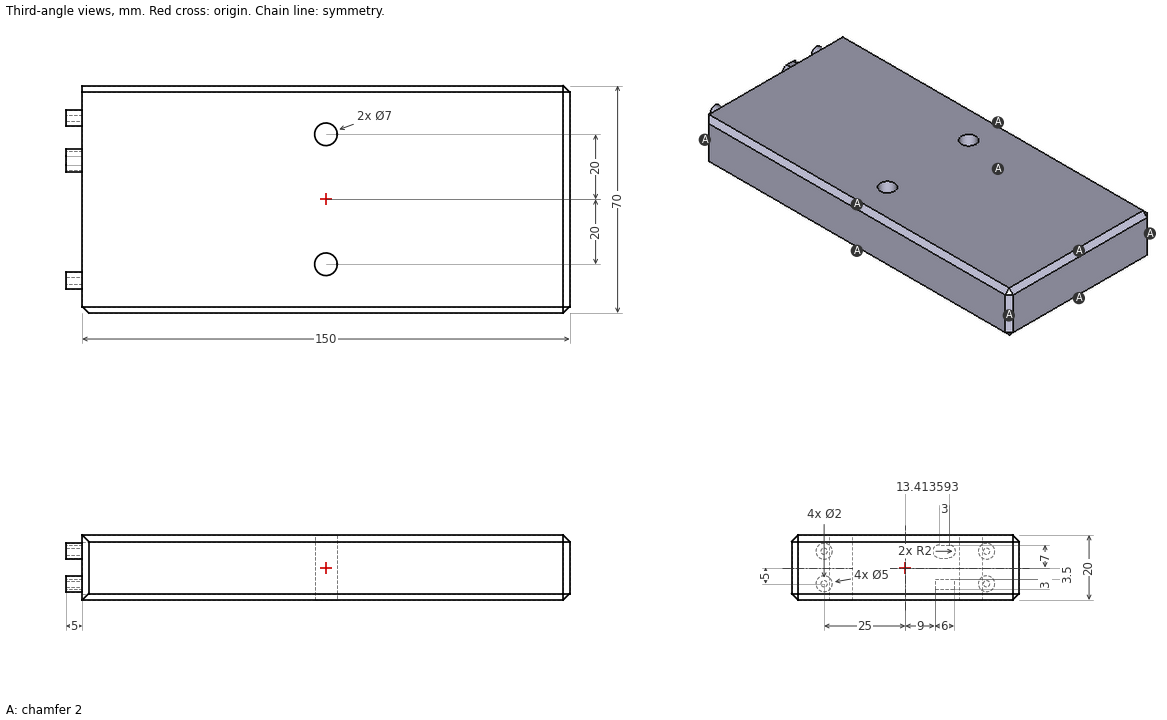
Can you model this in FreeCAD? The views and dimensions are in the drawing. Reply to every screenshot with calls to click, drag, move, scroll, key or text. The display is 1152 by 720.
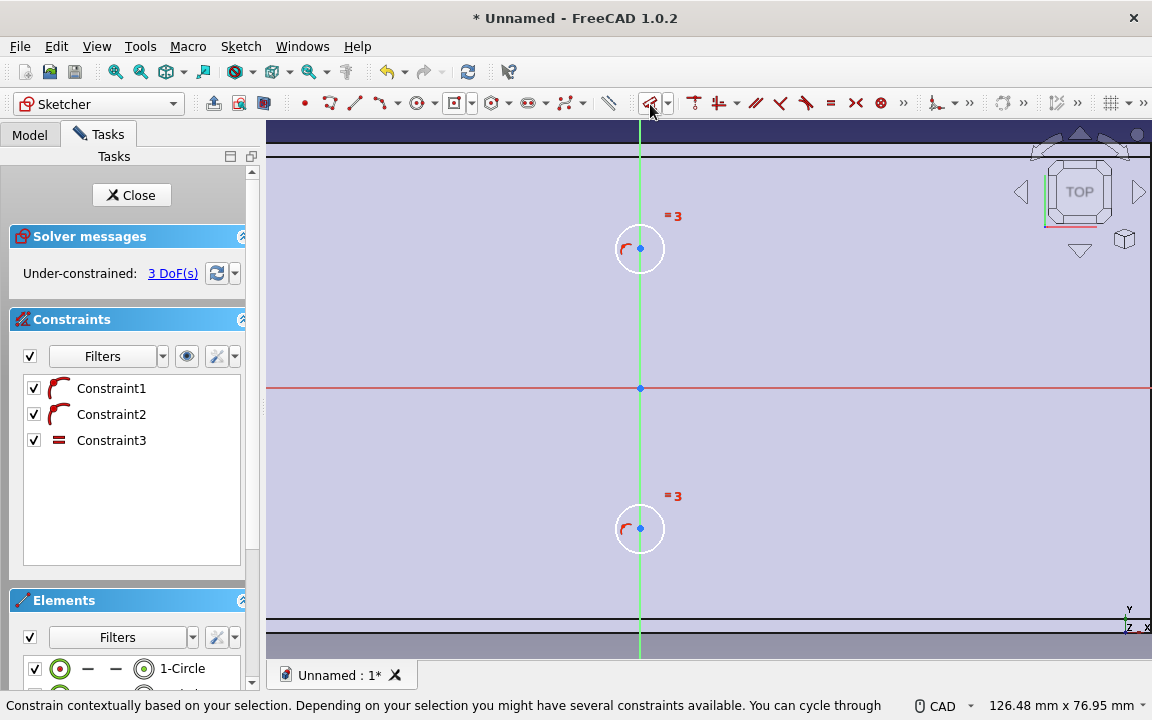
click(657, 232)
click(680, 209)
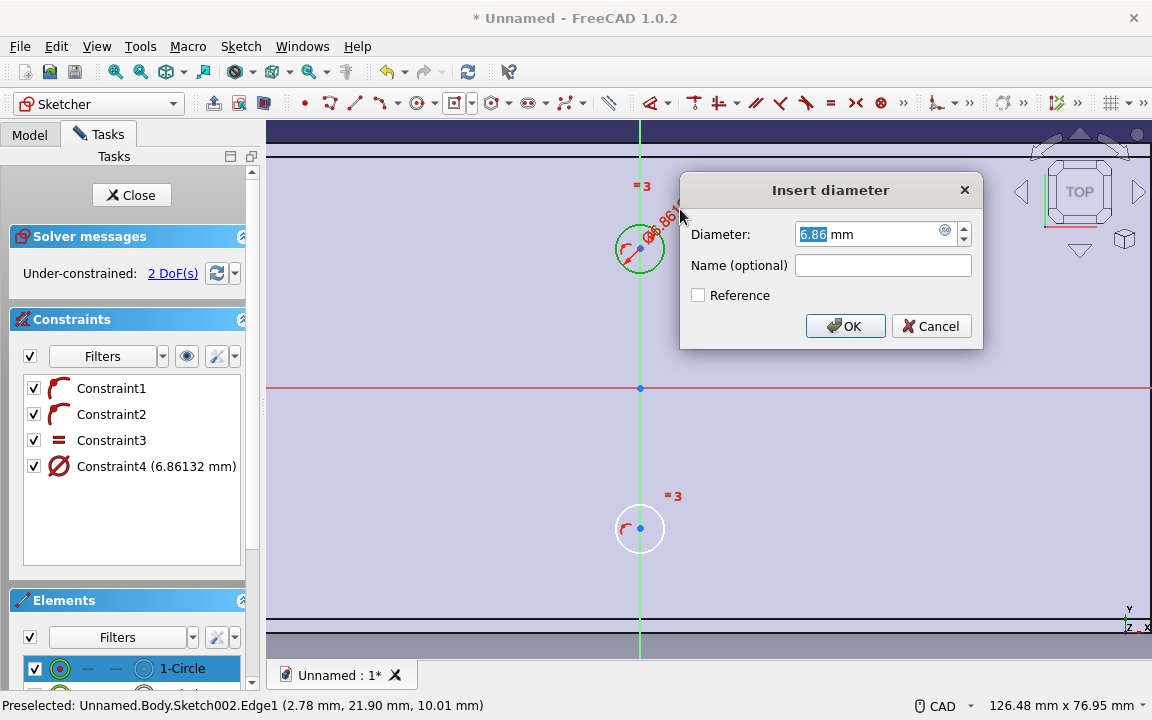
text(7)
key(Return)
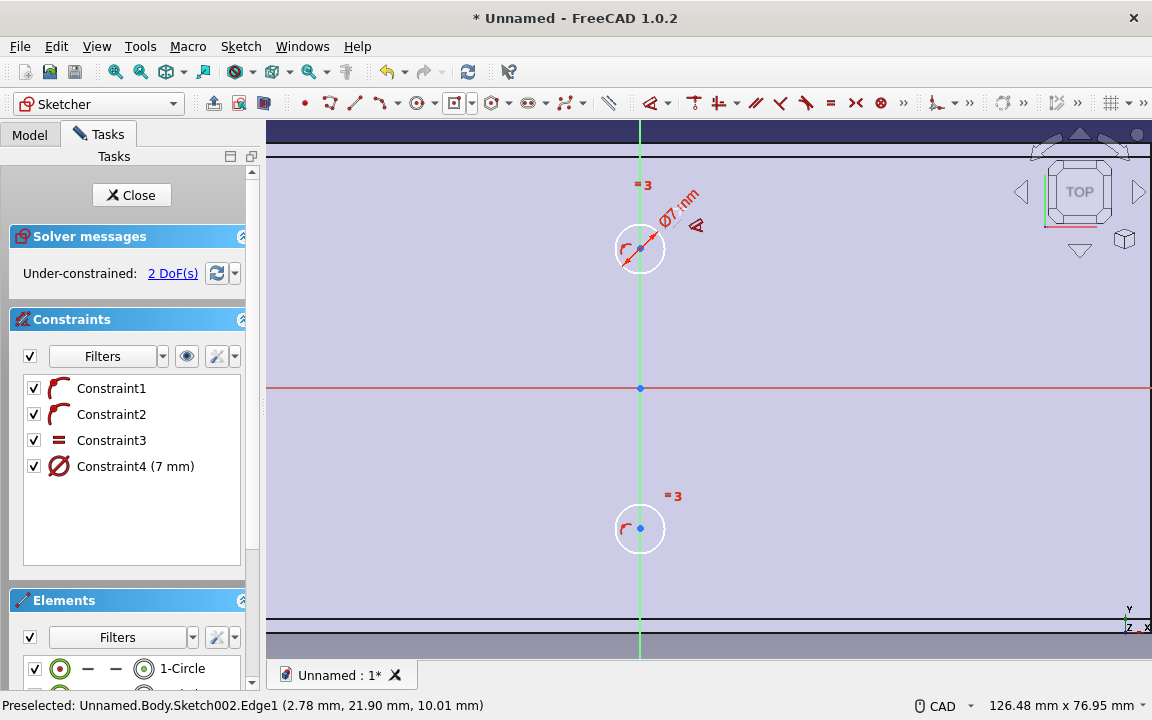
click(640, 249)
click(674, 319)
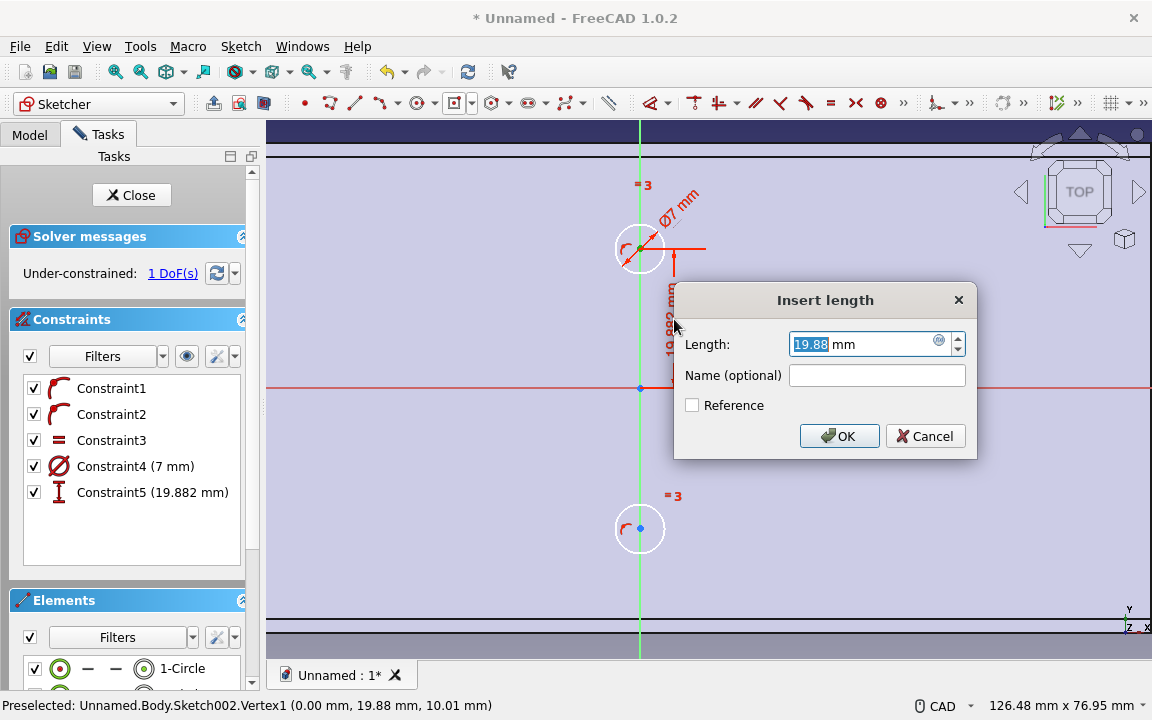
text(20)
key(Return)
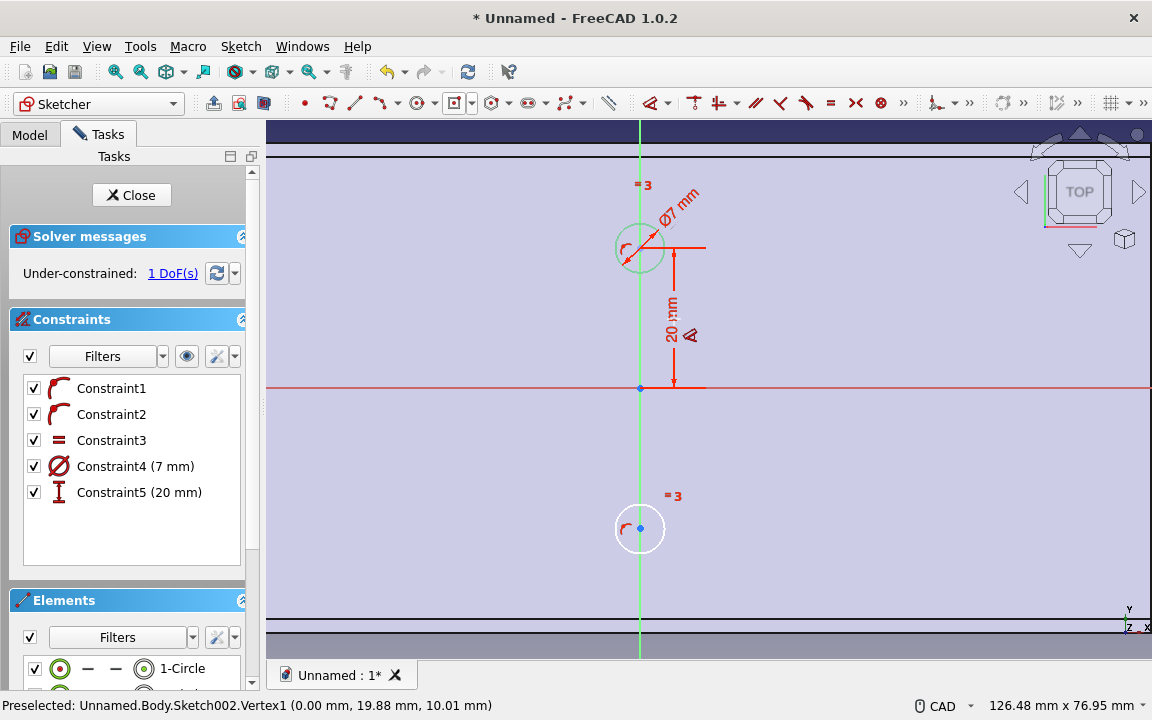
click(640, 529)
click(674, 459)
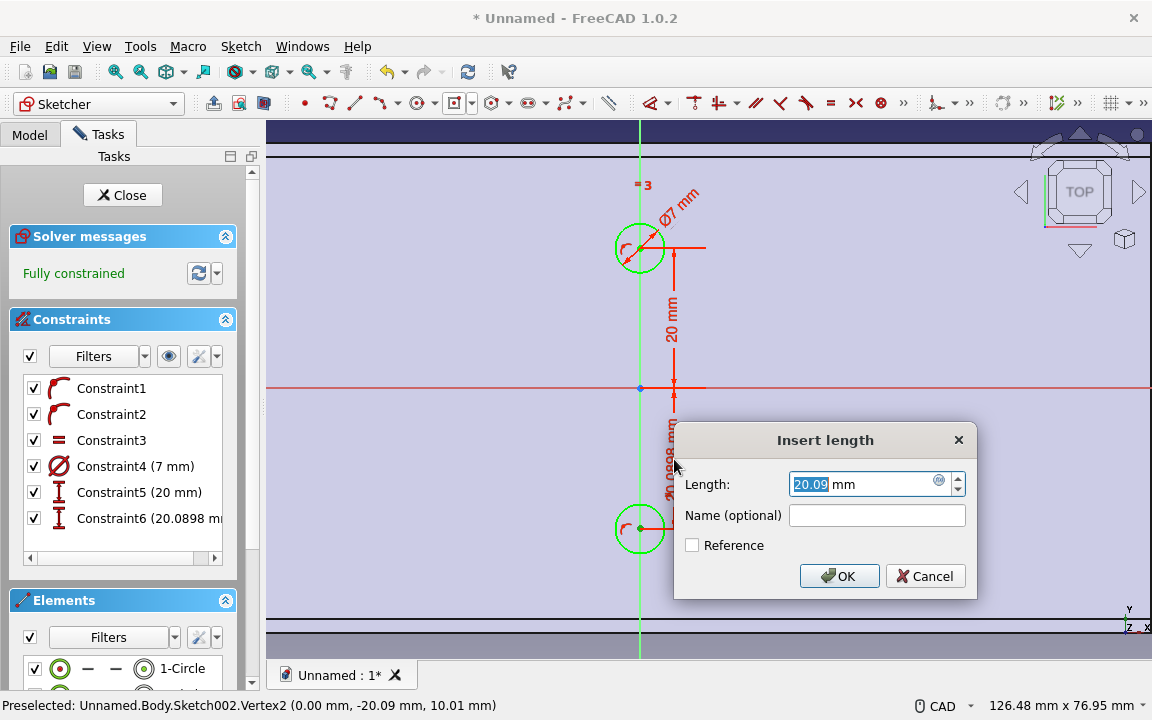
text(20)
key(Return)
key(Escape)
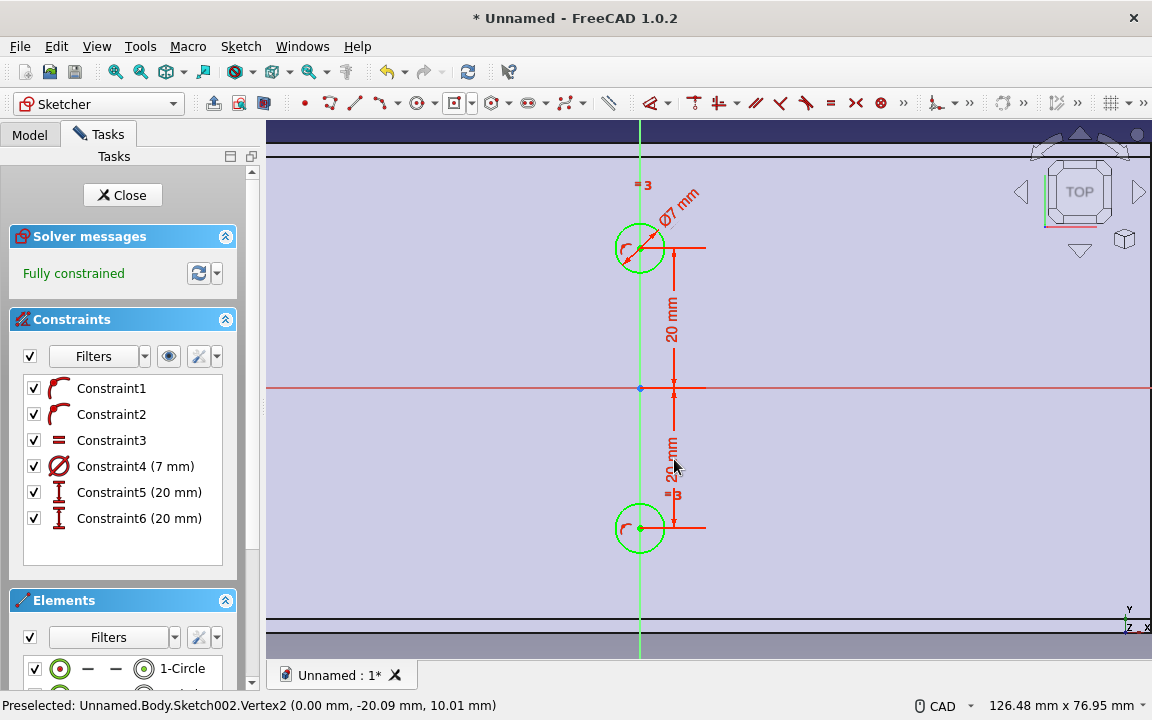
click(123, 195)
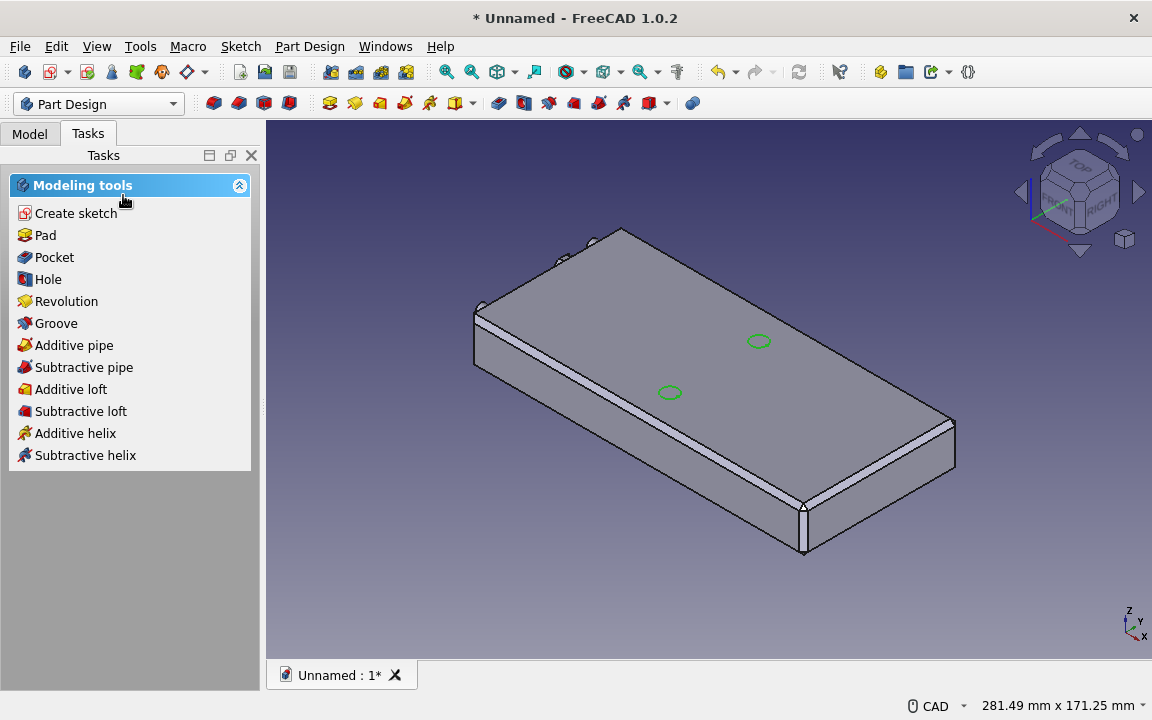
click(499, 104)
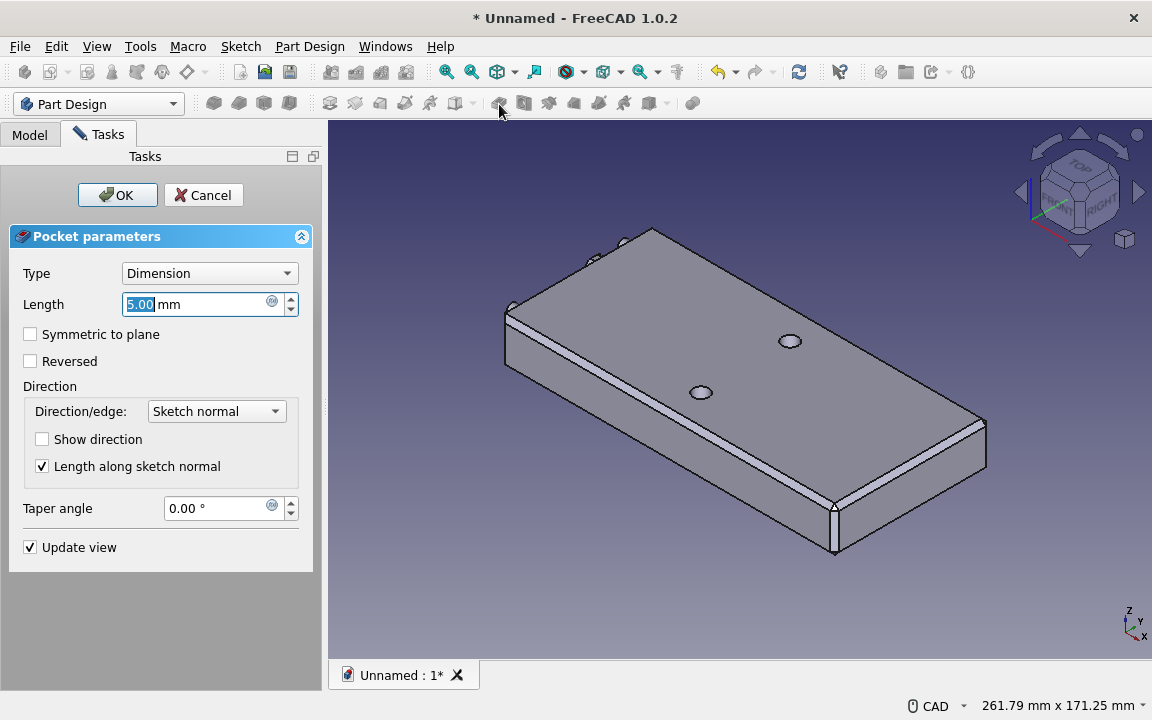
click(210, 274)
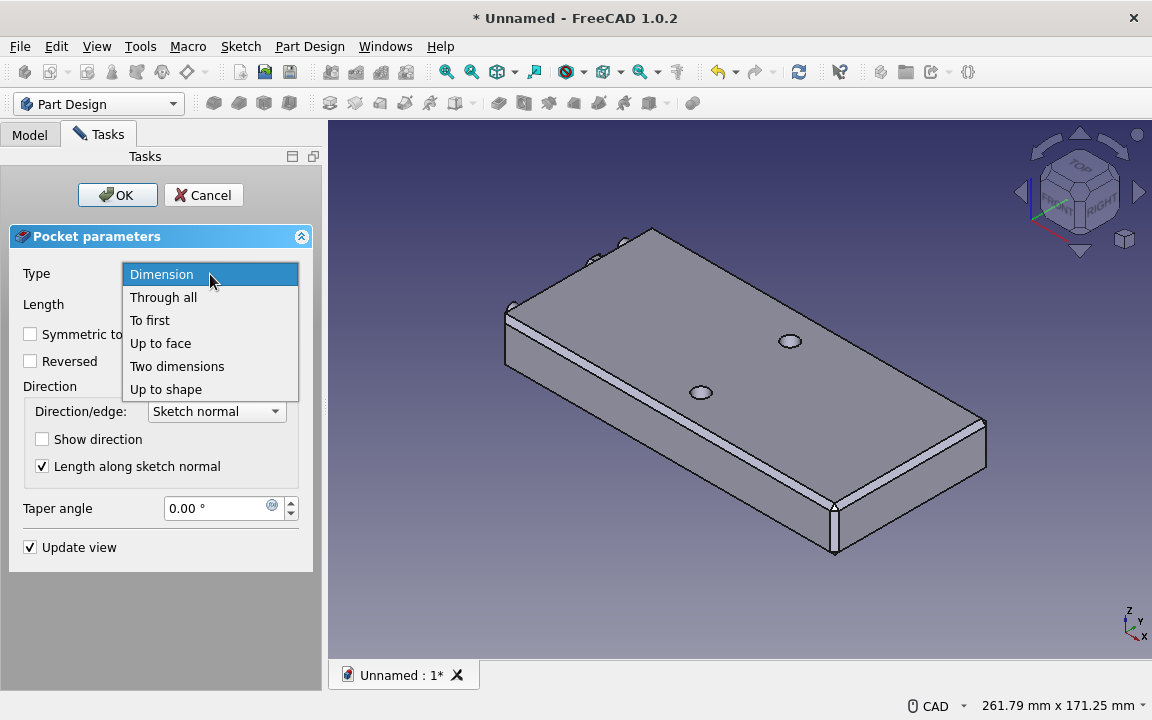
click(208, 298)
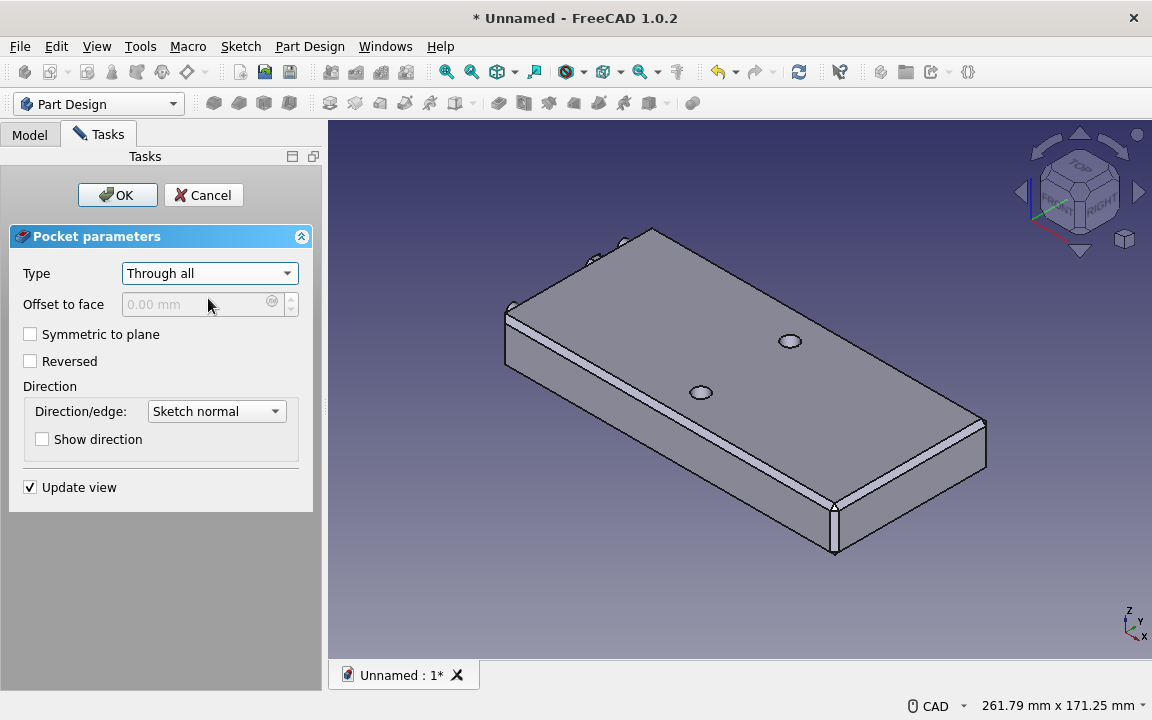
click(118, 195)